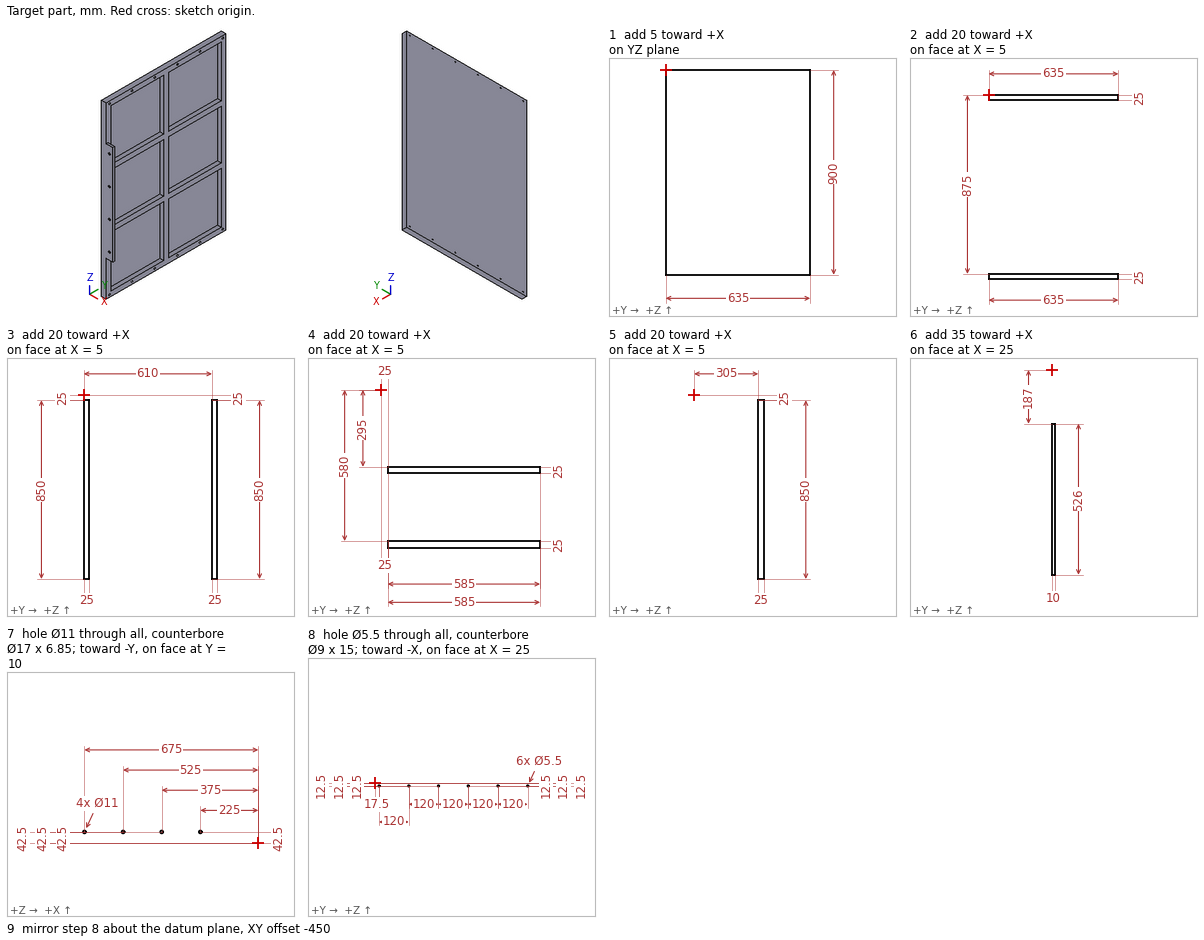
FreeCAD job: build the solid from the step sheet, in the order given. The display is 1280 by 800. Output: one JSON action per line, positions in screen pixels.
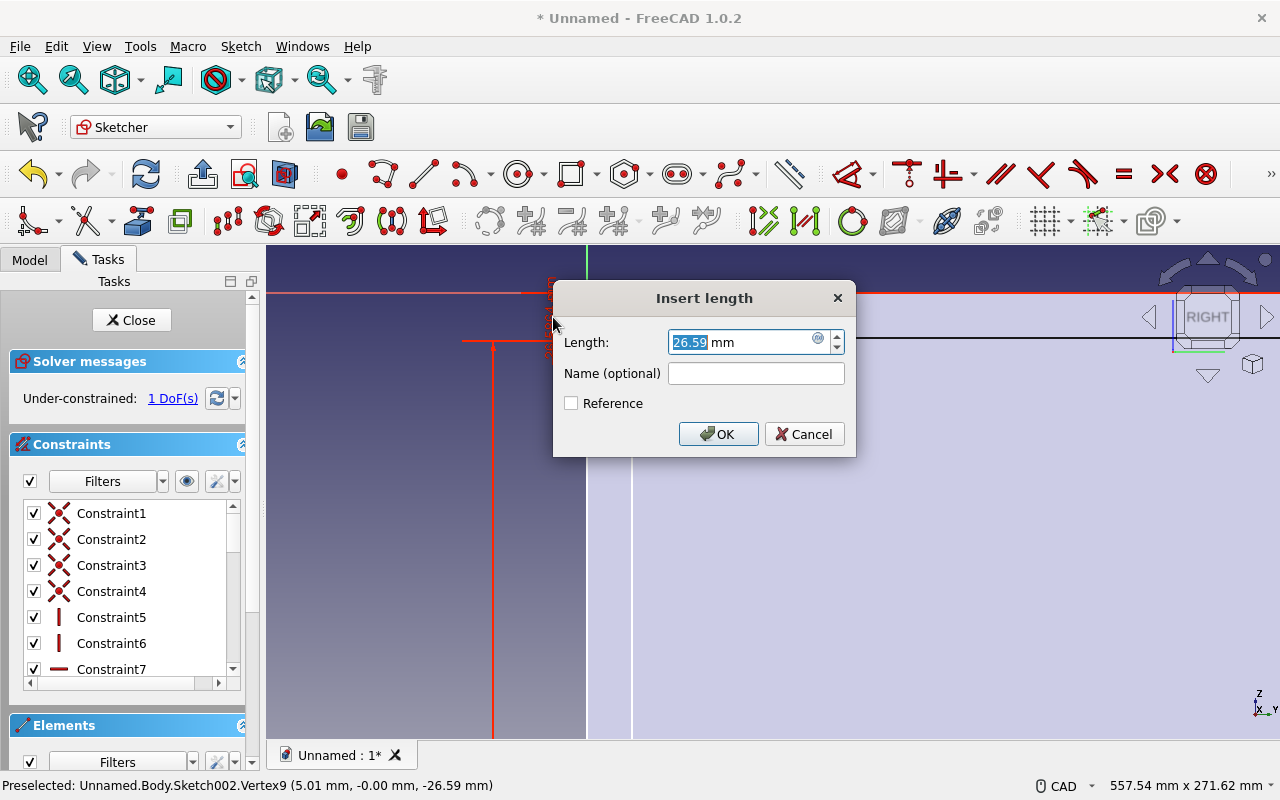
{"action": "type", "text": "25"}
{"action": "key", "text": "Return"}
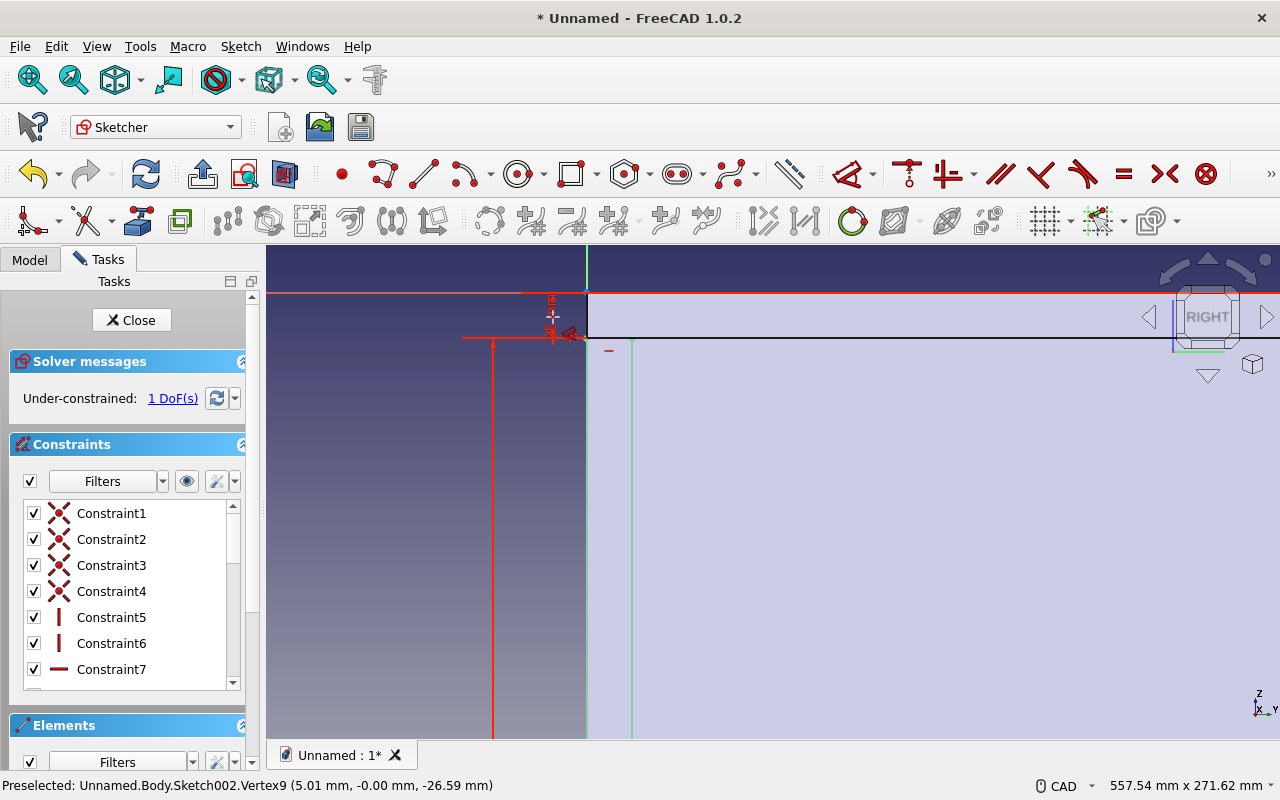
{"action": "scroll", "coordinate": [588, 341], "scroll_direction": "down", "scroll_amount": 8}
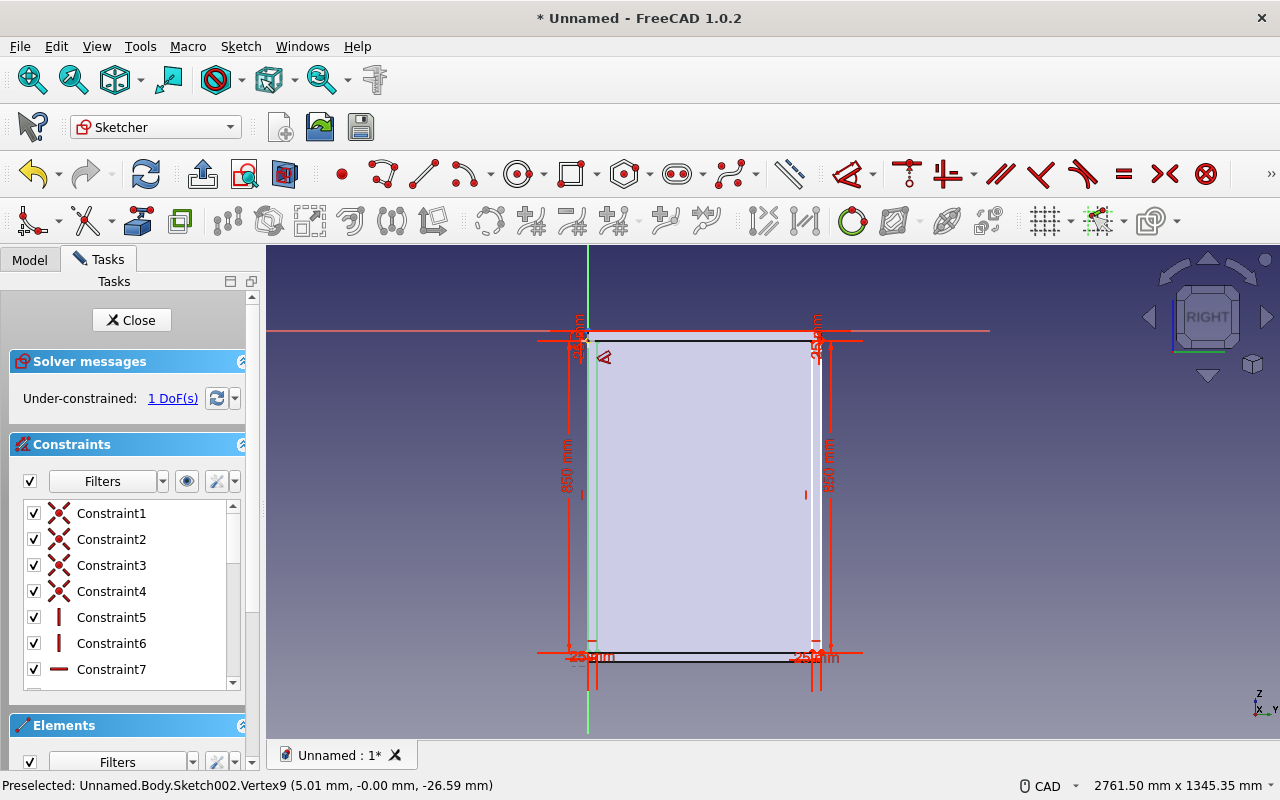
{"action": "scroll", "coordinate": [812, 341], "scroll_direction": "up", "scroll_amount": 2}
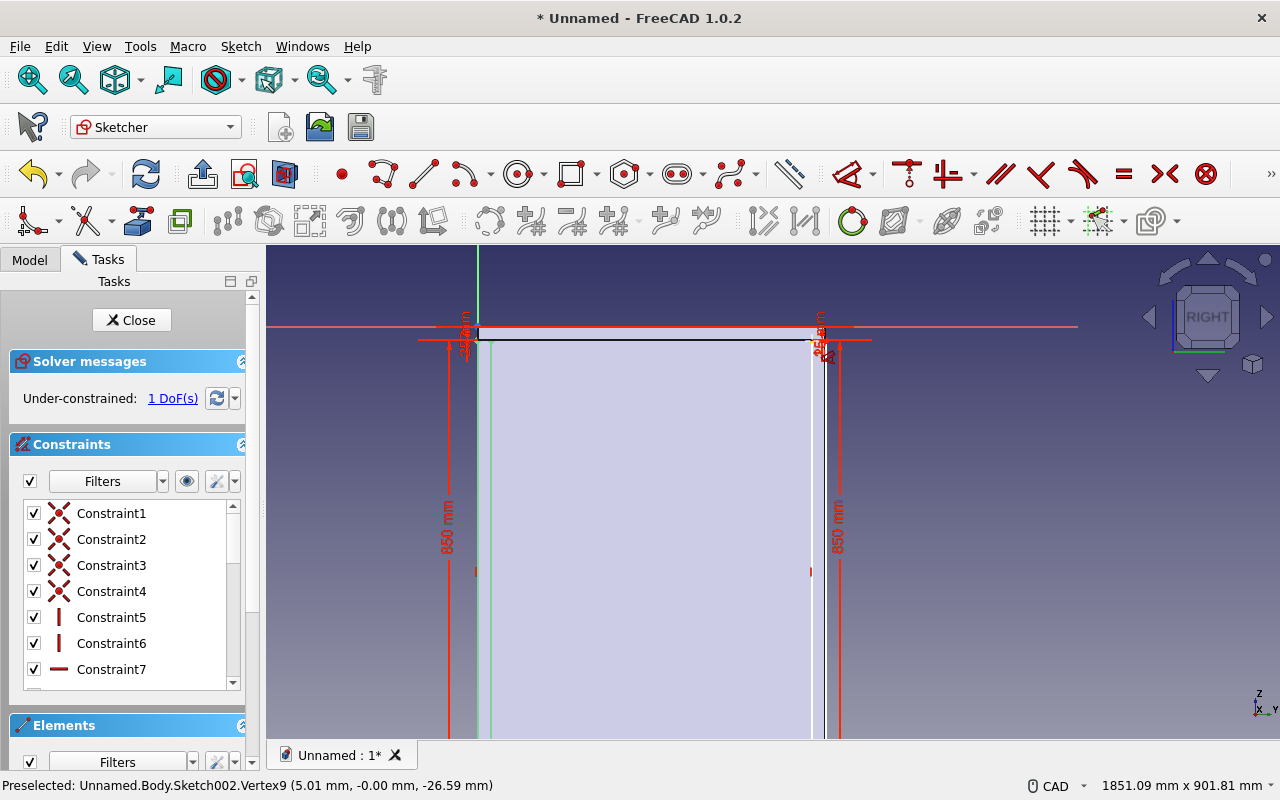
{"action": "left_click", "coordinate": [812, 340]}
{"action": "left_click", "coordinate": [645, 293]}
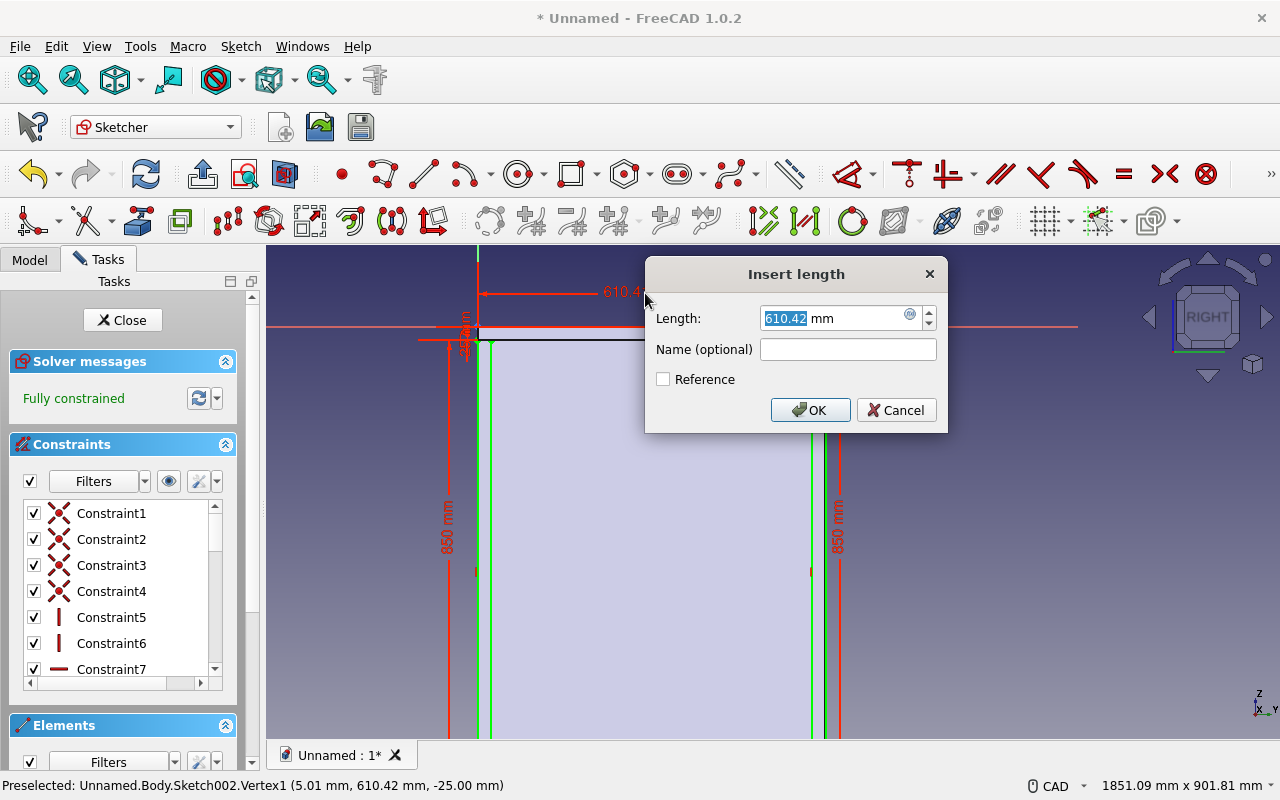
{"action": "type", "text": "610"}
{"action": "key", "text": "Return"}
{"action": "key", "text": "Escape"}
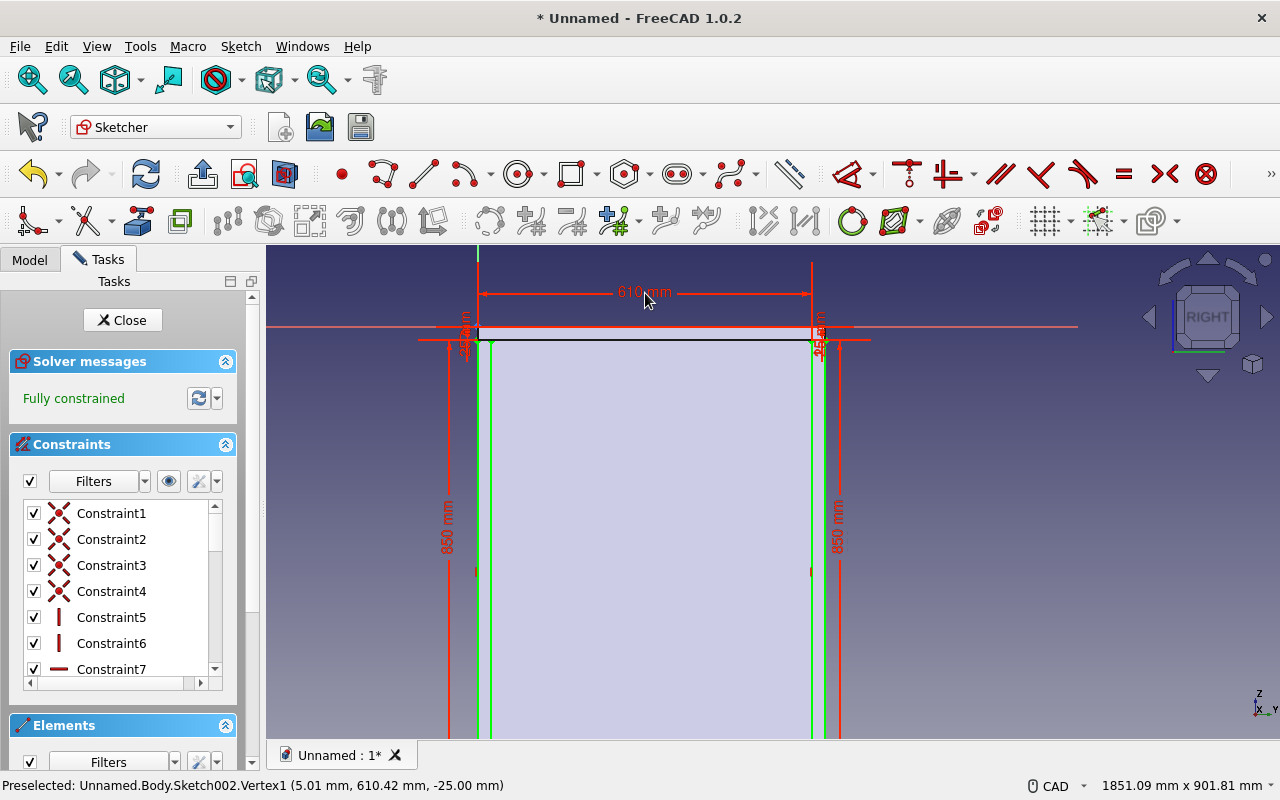
{"action": "left_click", "coordinate": [123, 320]}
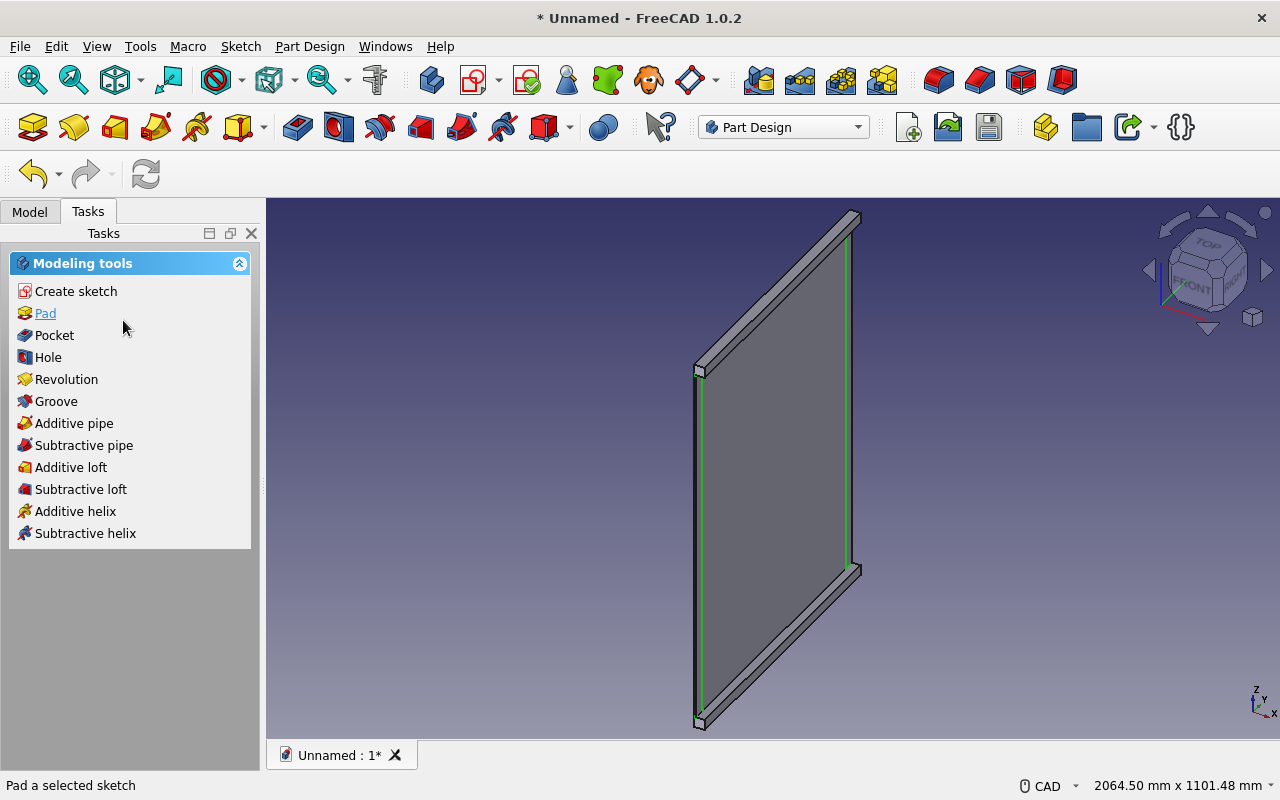
{"action": "left_click", "coordinate": [33, 128]}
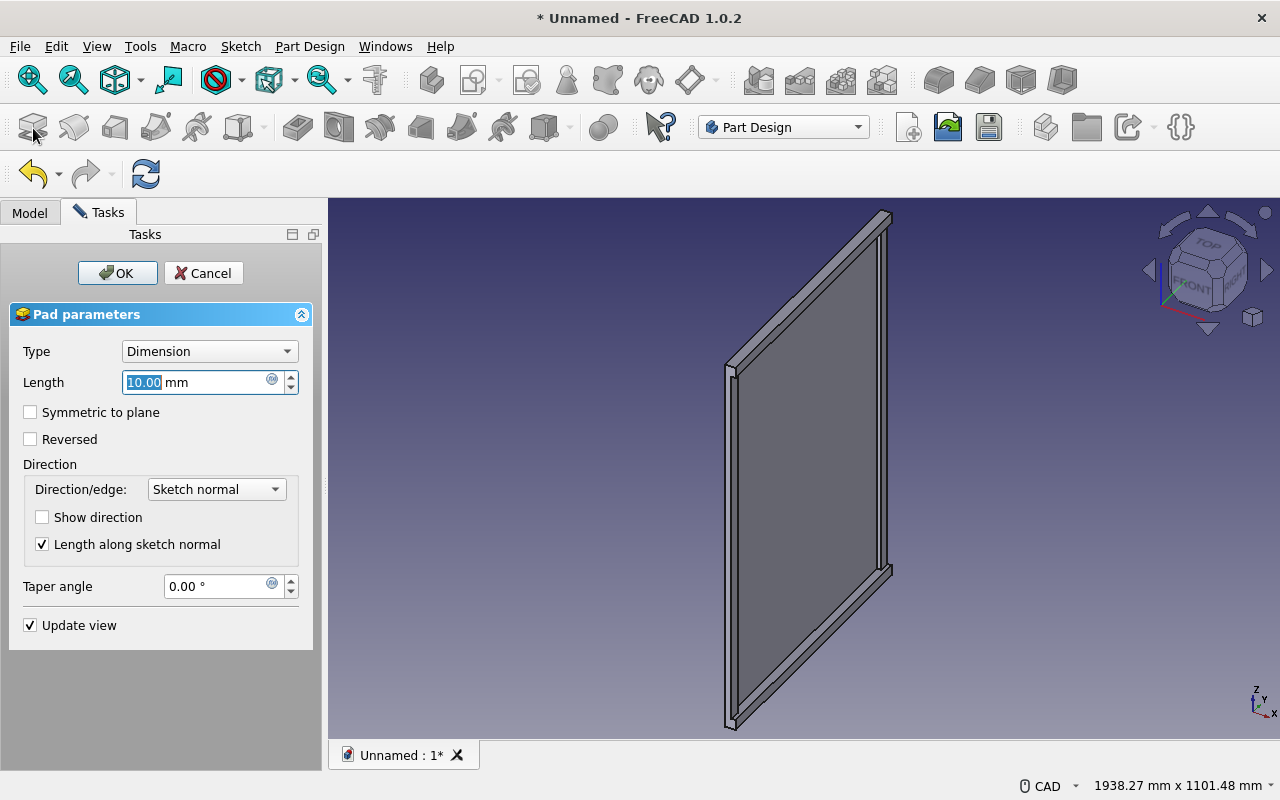
{"action": "type", "text": "20"}
{"action": "key", "text": "Tab"}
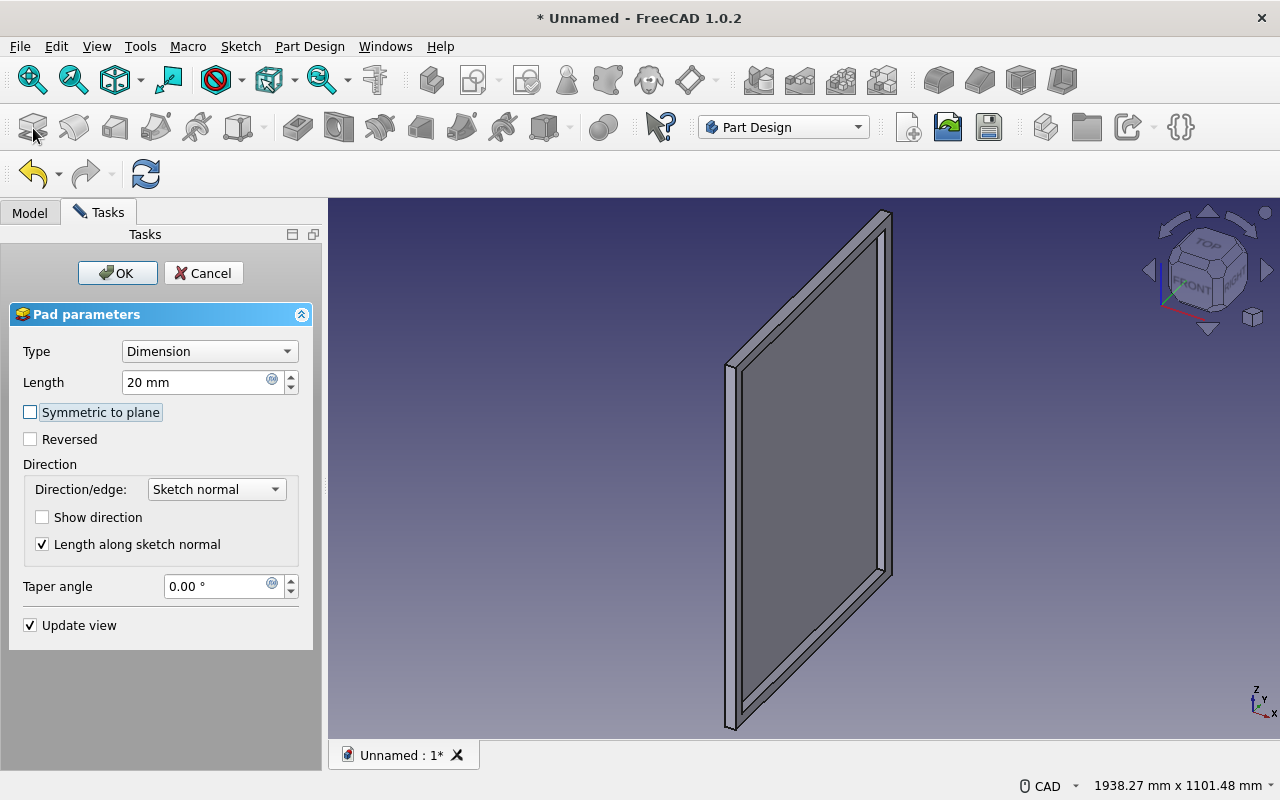
{"action": "left_click", "coordinate": [118, 273]}